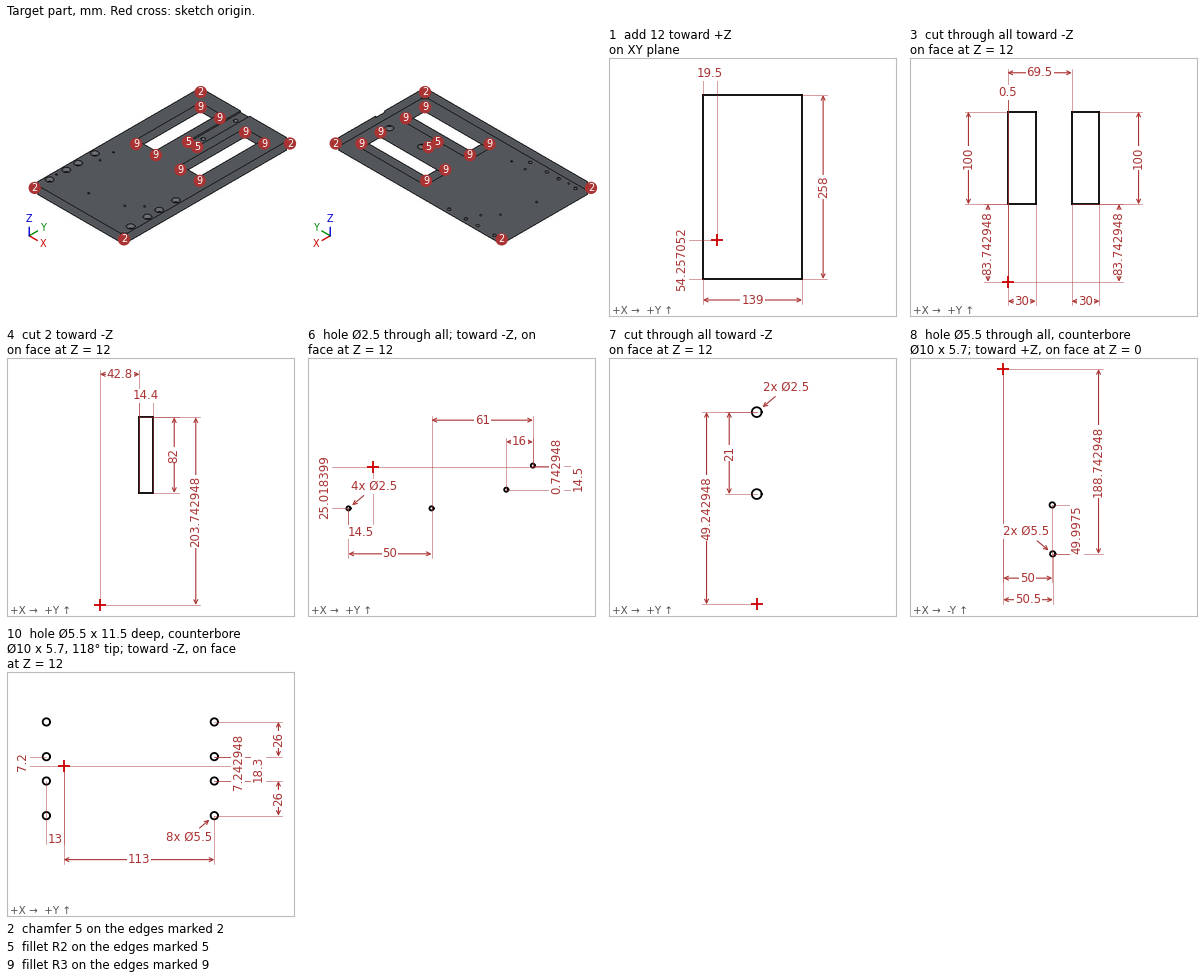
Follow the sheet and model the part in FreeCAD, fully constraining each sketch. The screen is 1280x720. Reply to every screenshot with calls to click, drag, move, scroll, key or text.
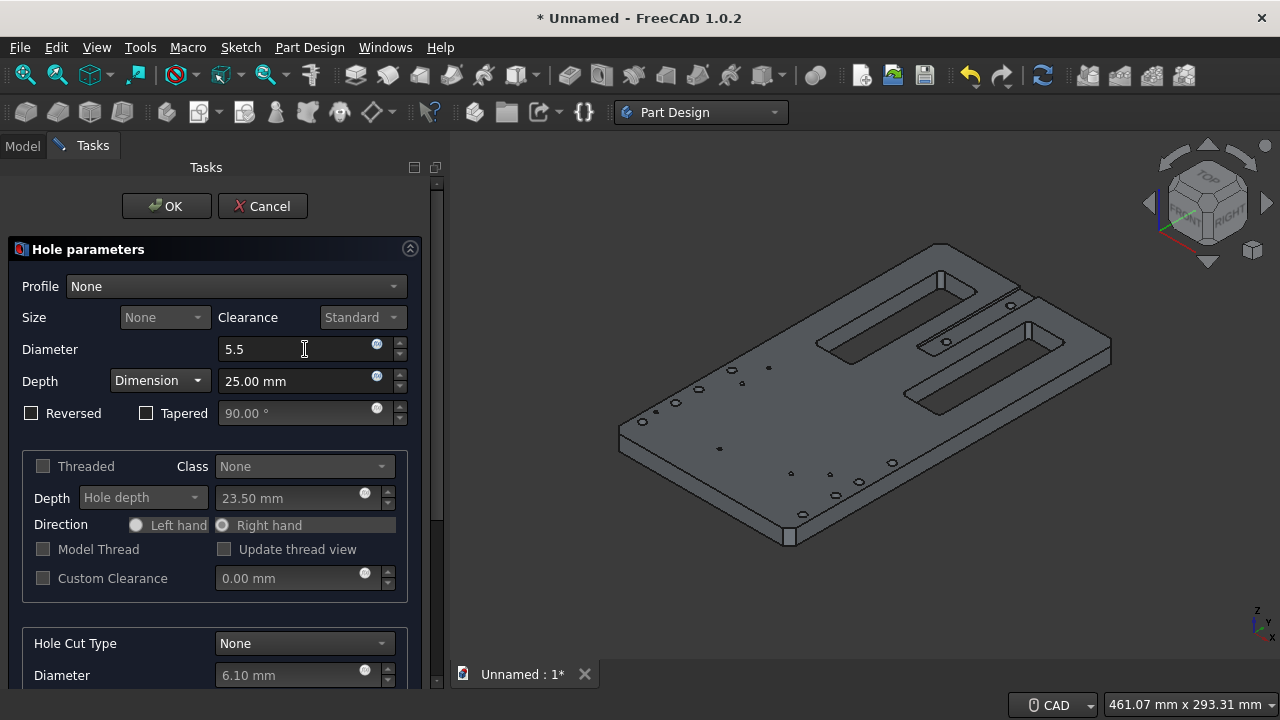
triple_click(305, 381)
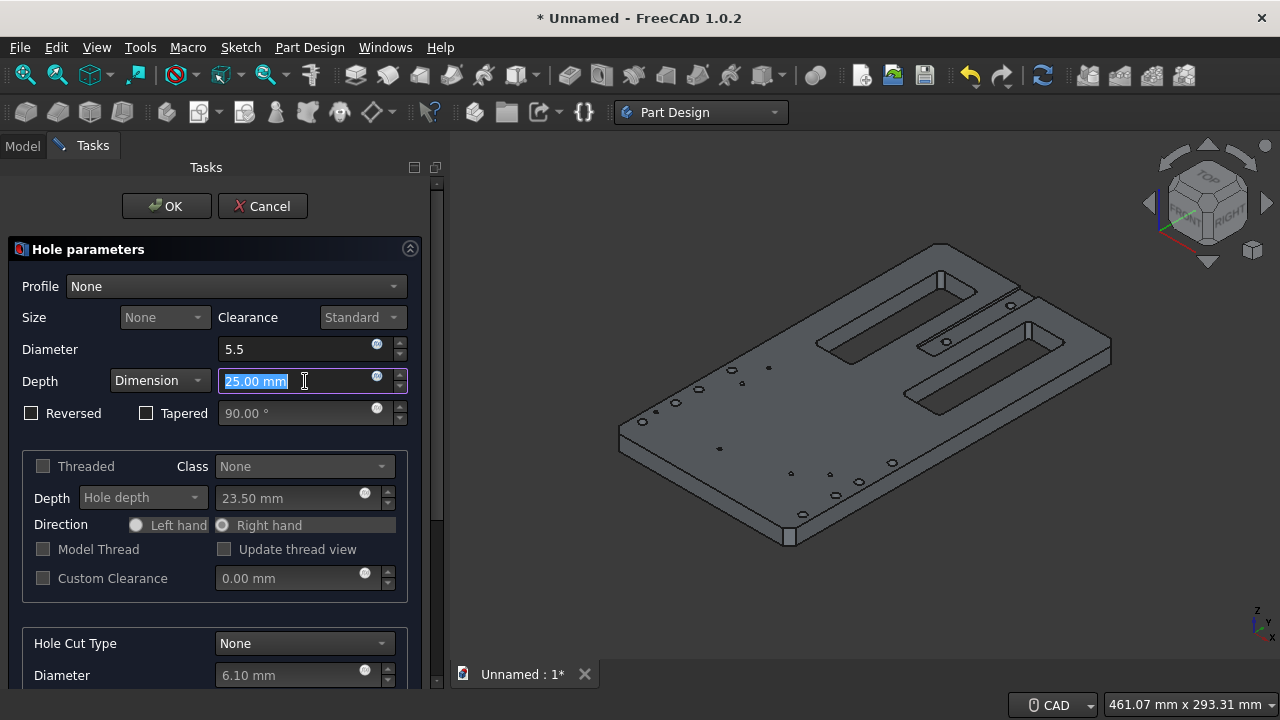
text(11.5)
key(Tab)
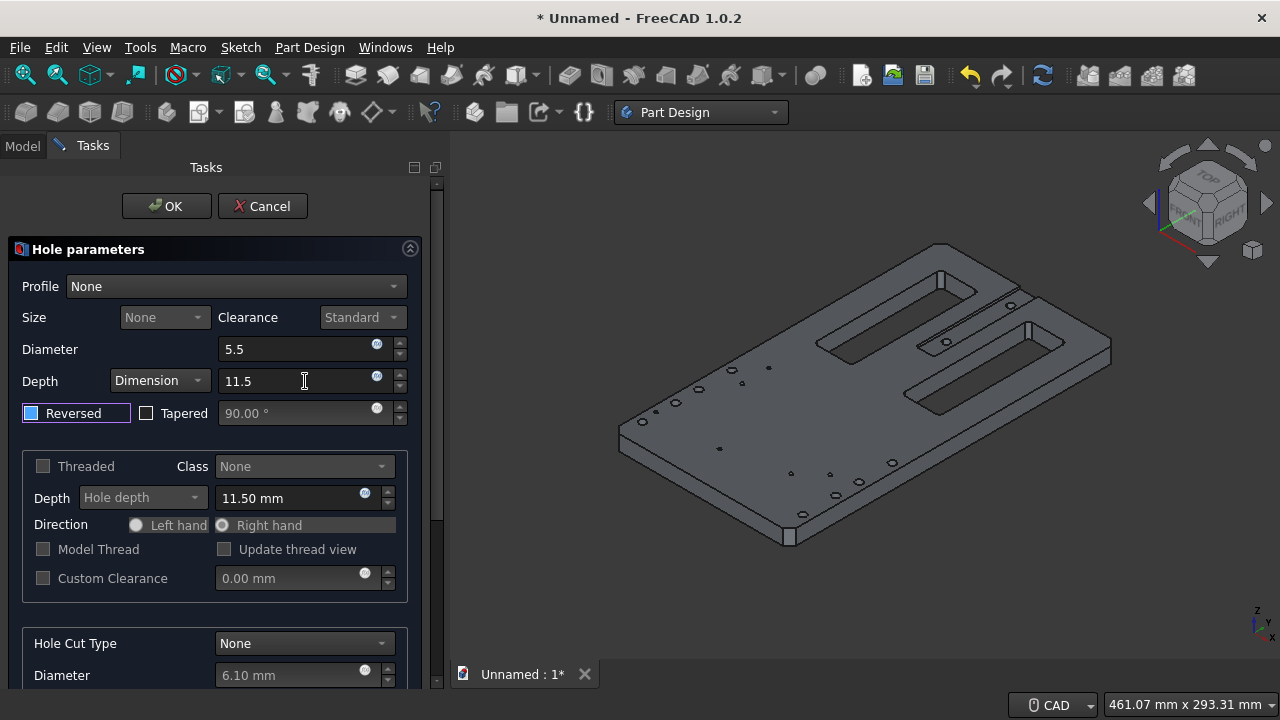
click(306, 644)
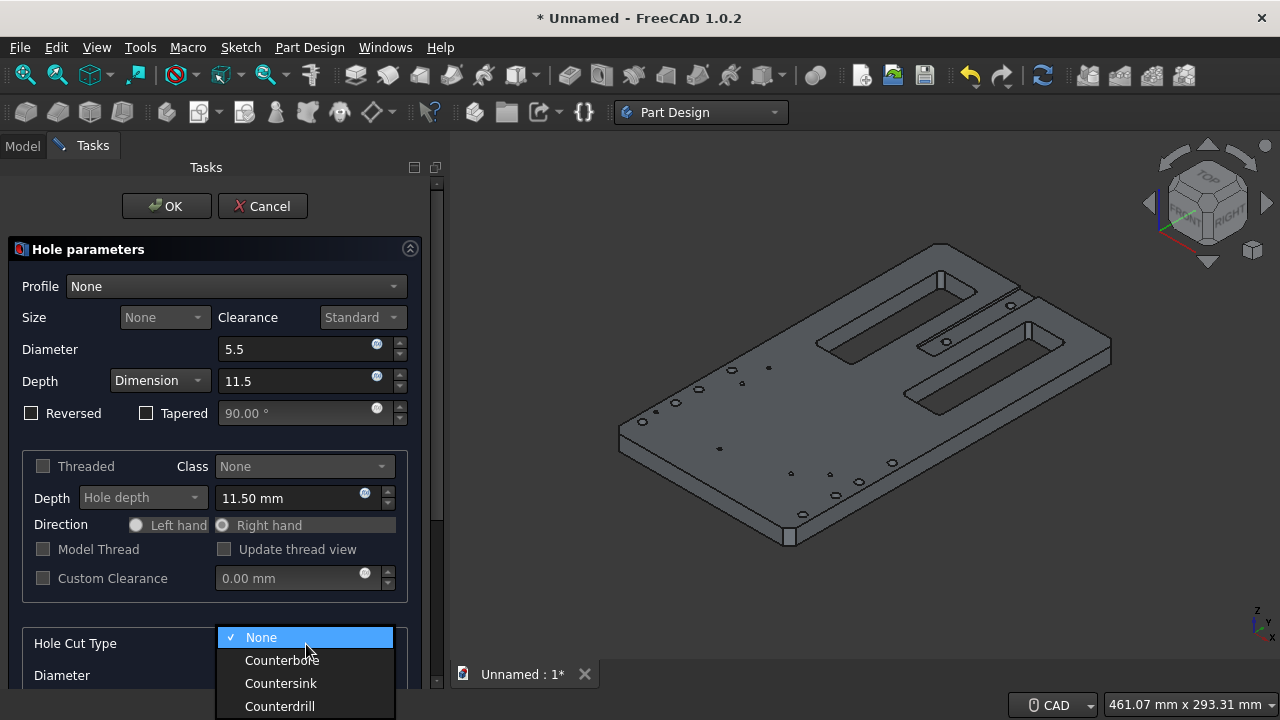
click(304, 660)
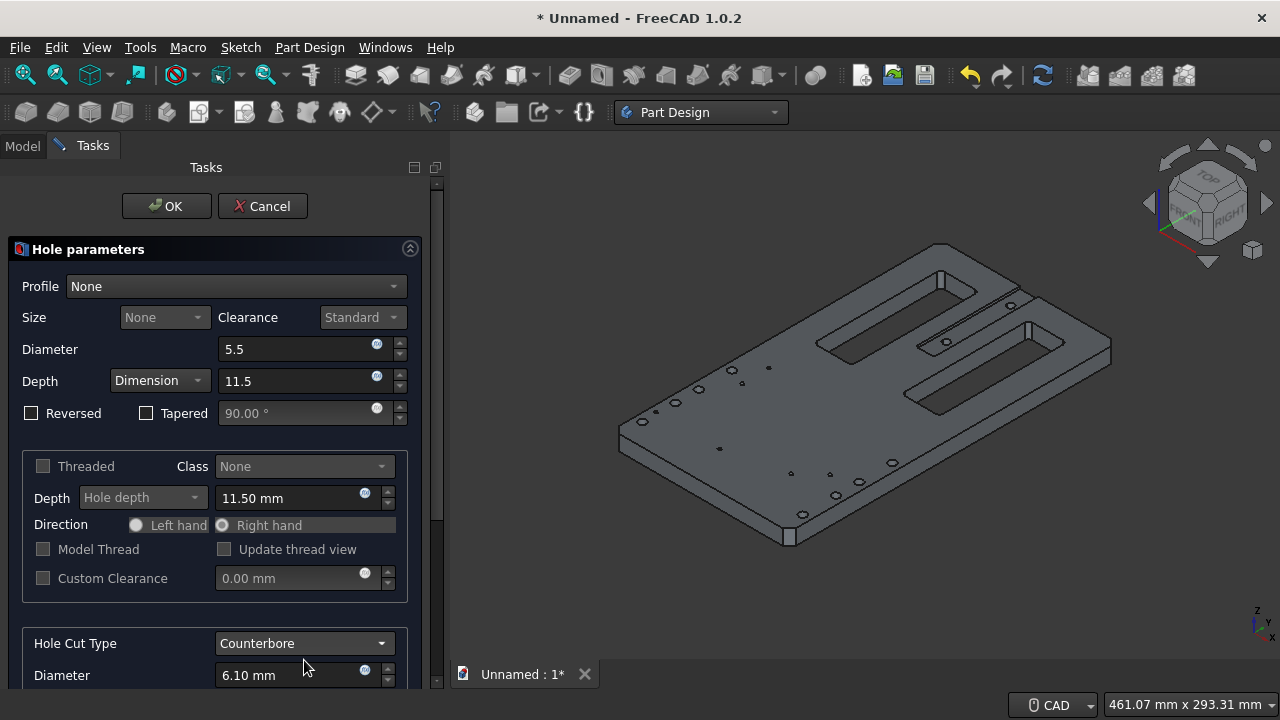
triple_click(298, 675)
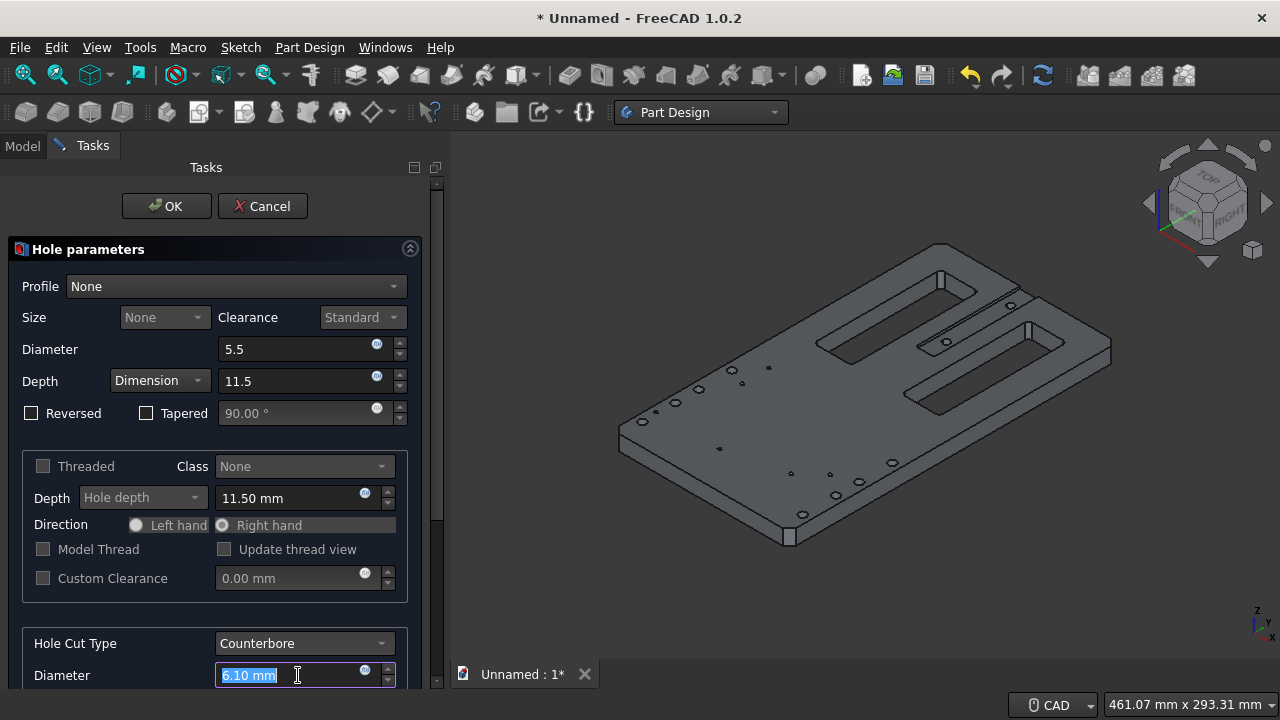
text(10)
key(Tab)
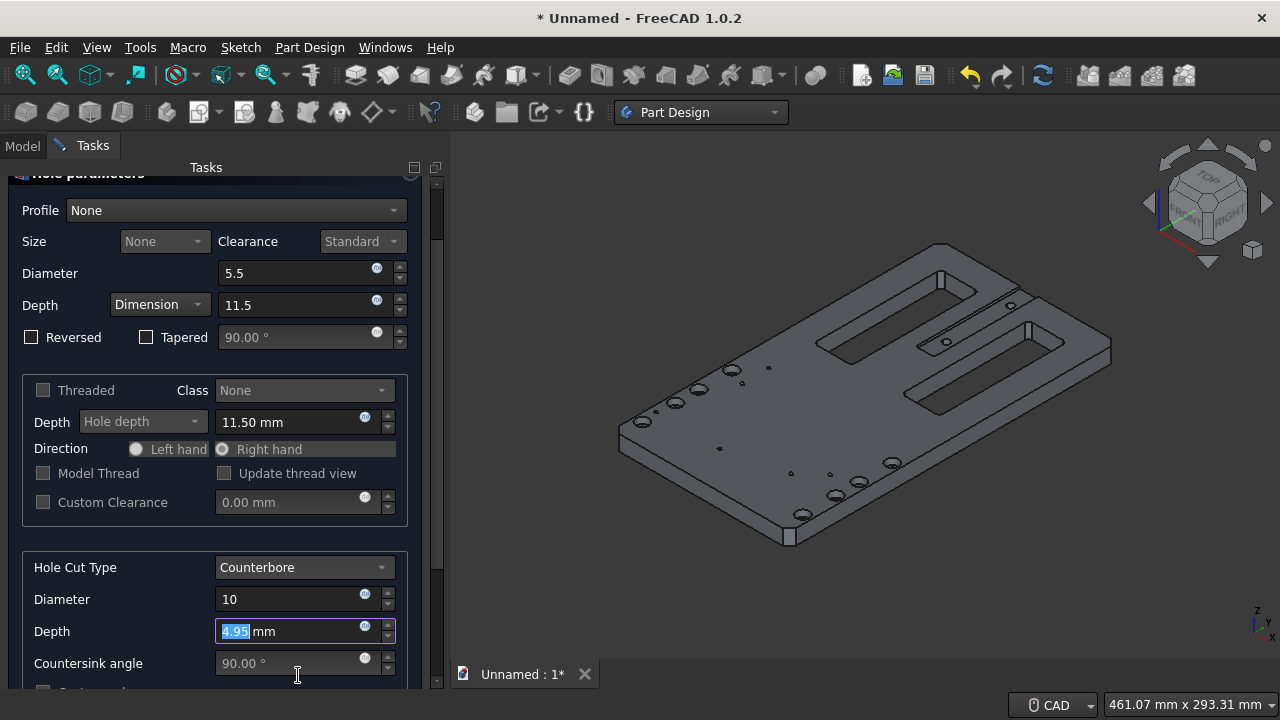
text(5.7)
key(Tab)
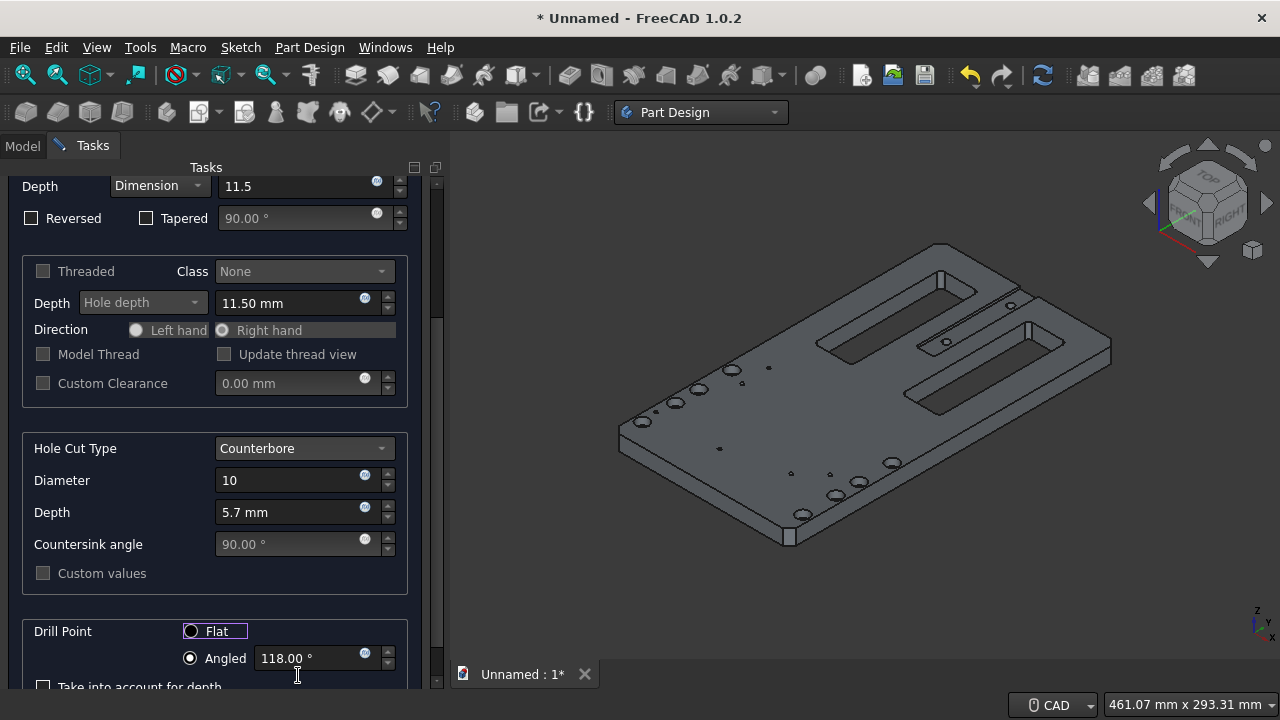
scroll(437, 432, up, 4)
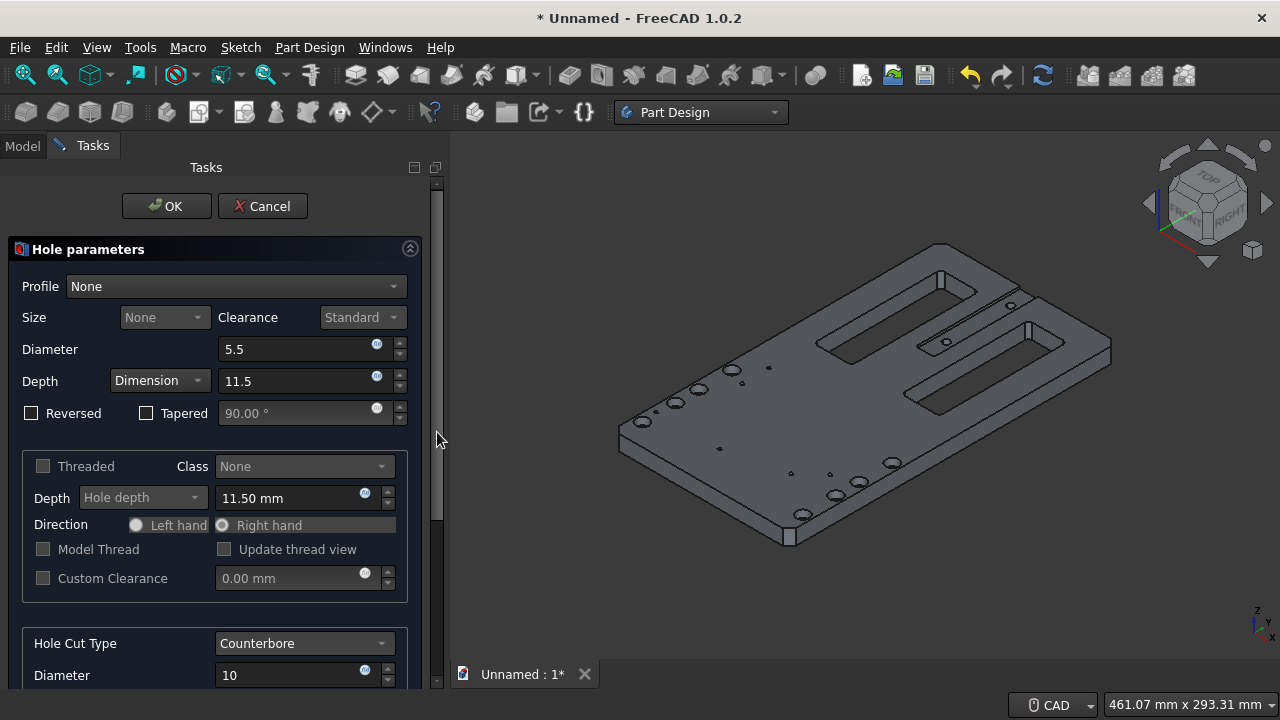
click(167, 206)